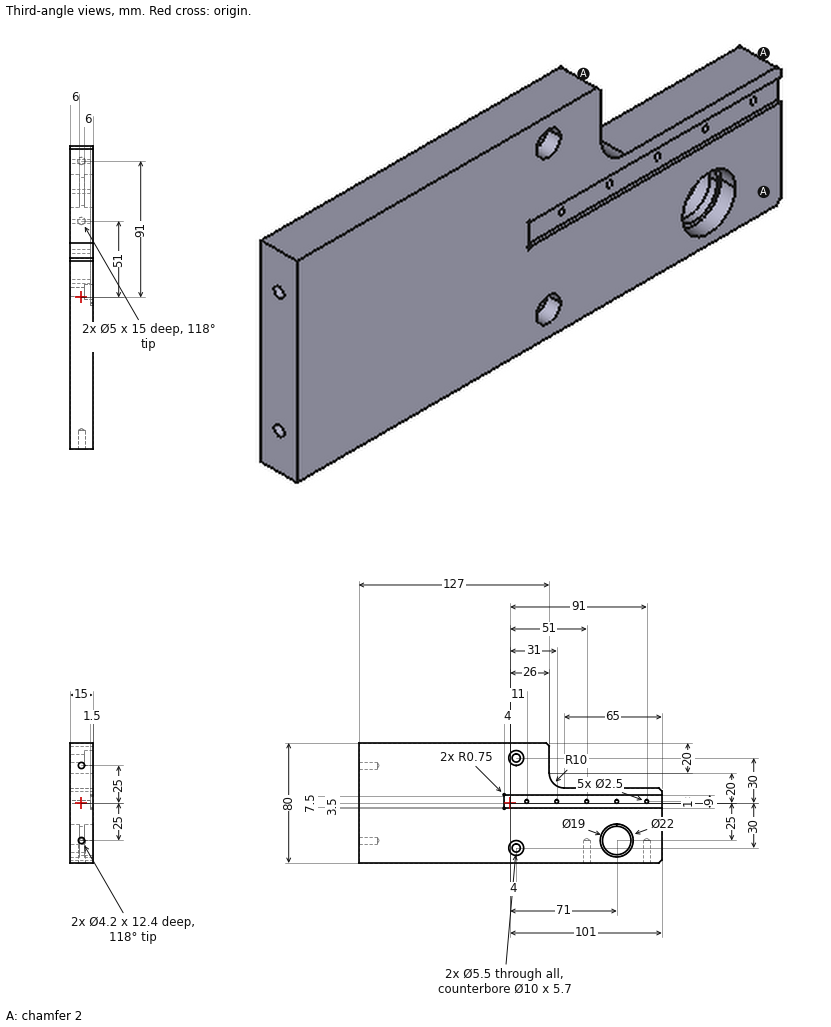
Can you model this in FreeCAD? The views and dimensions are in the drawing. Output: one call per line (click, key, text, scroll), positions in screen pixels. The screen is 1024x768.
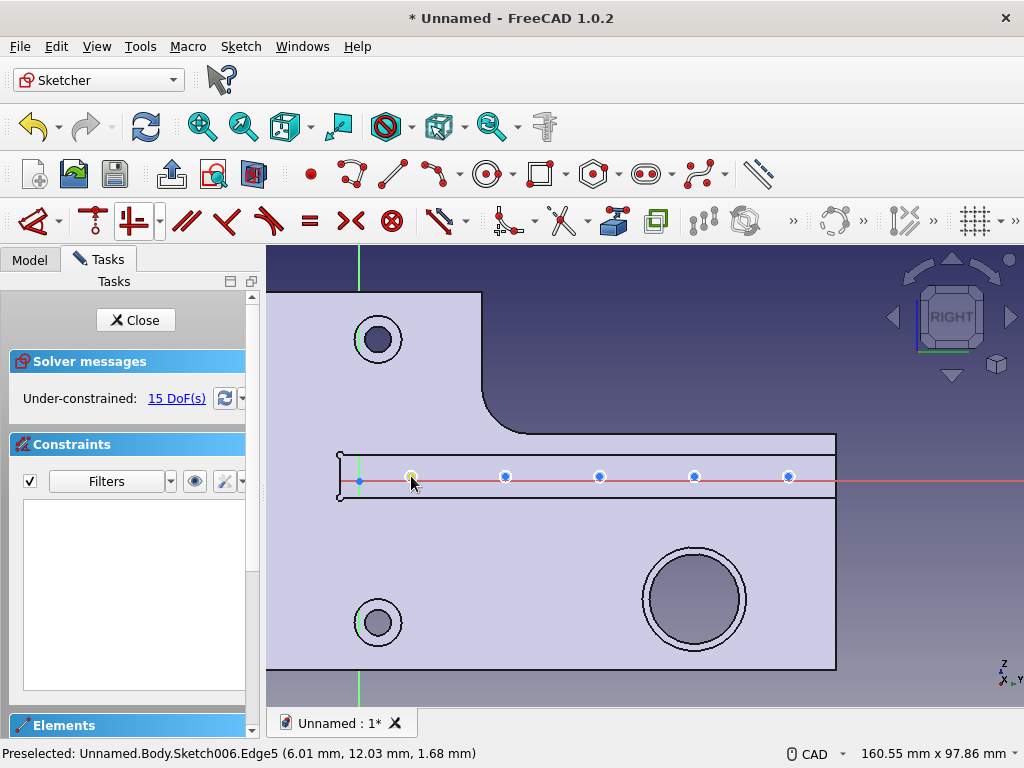
scroll(793, 472, up, 5)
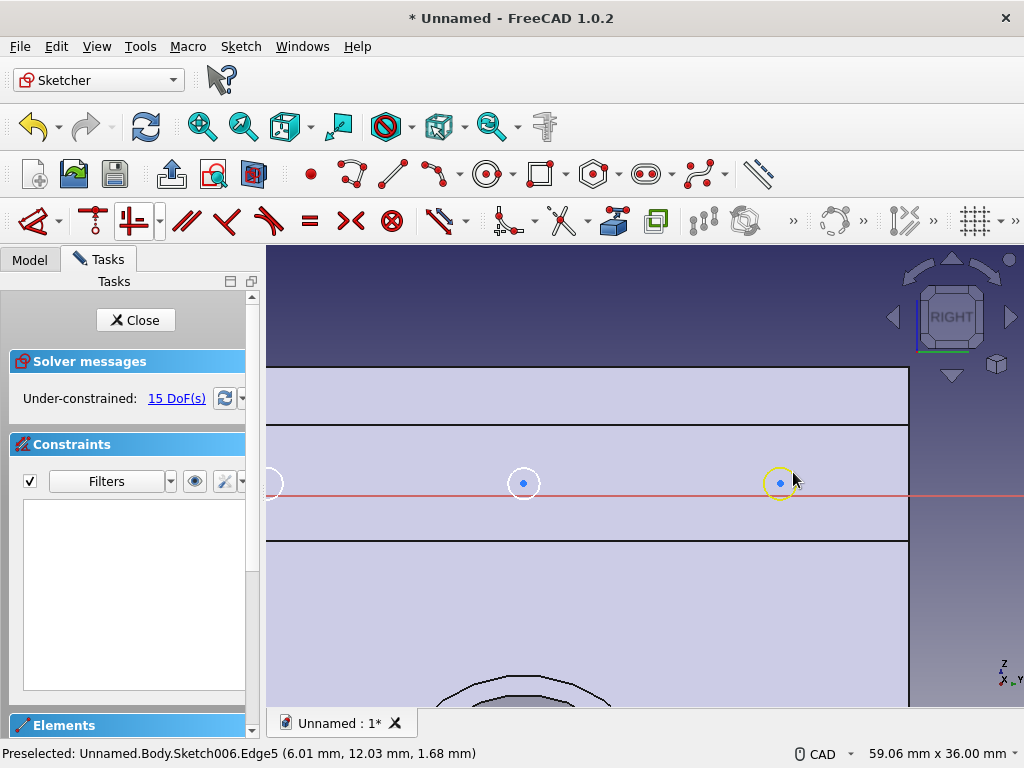
click(791, 472)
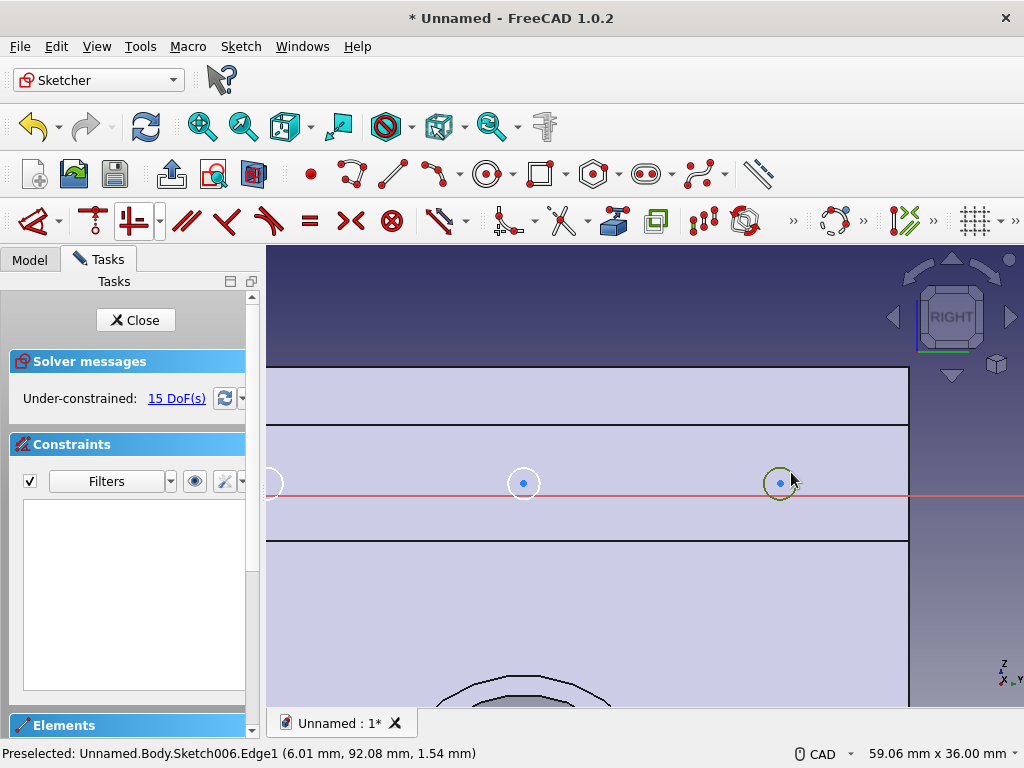
click(535, 473)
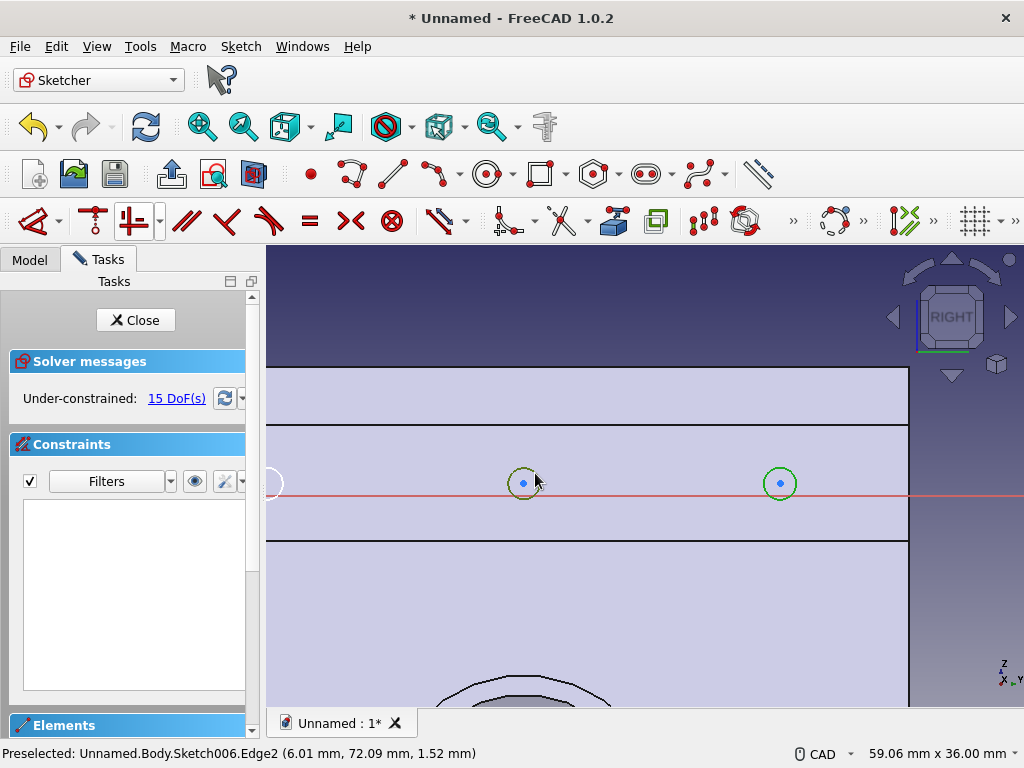
scroll(793, 472, down, 5)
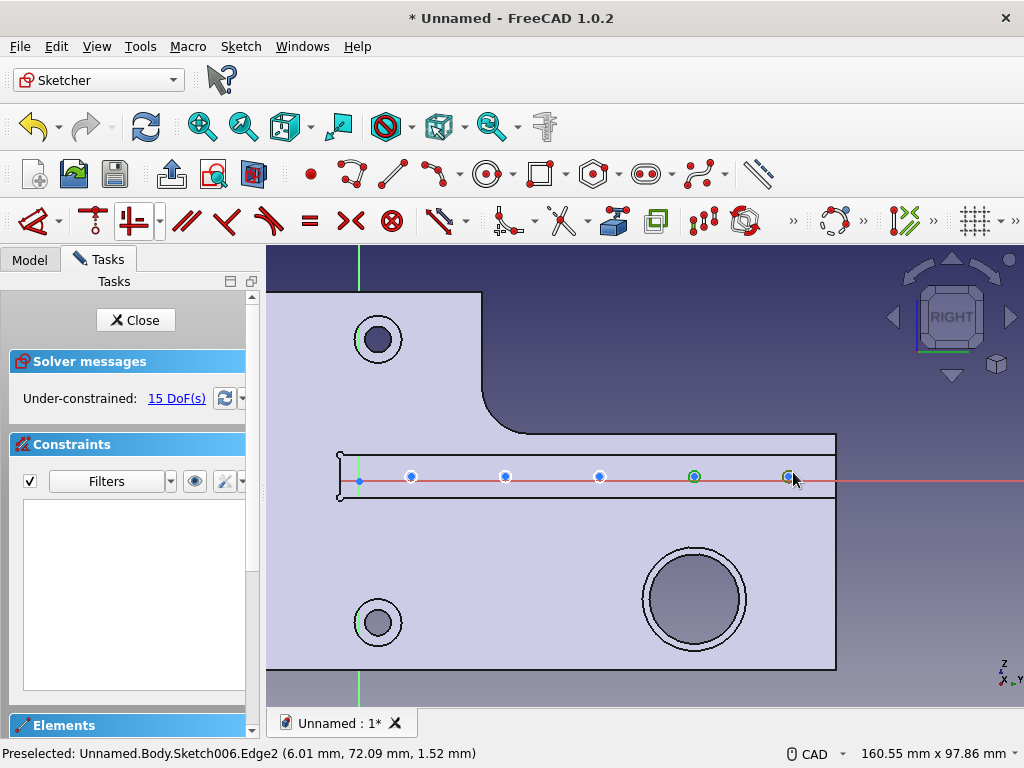
scroll(604, 472, up, 5)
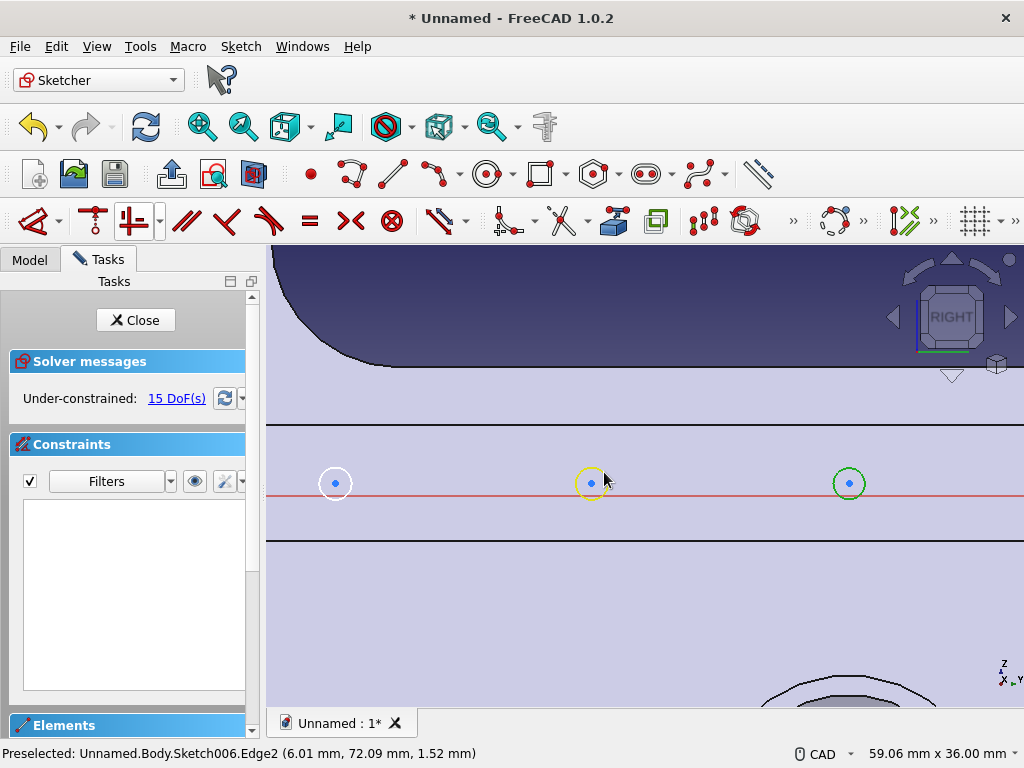
click(603, 472)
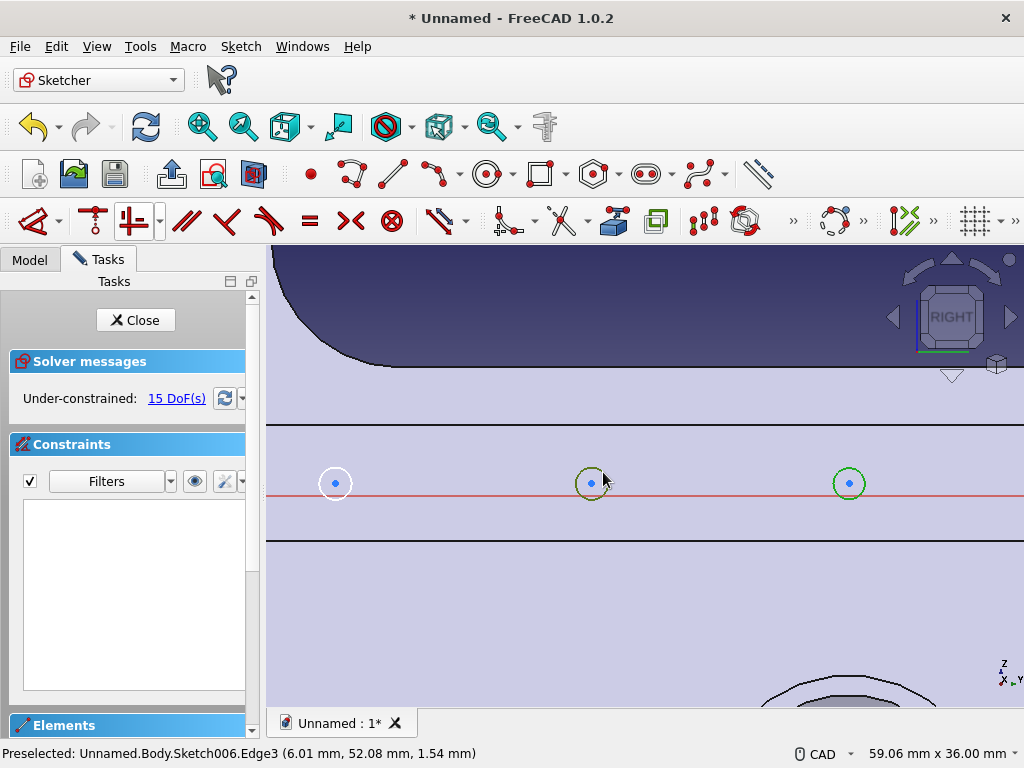
click(347, 472)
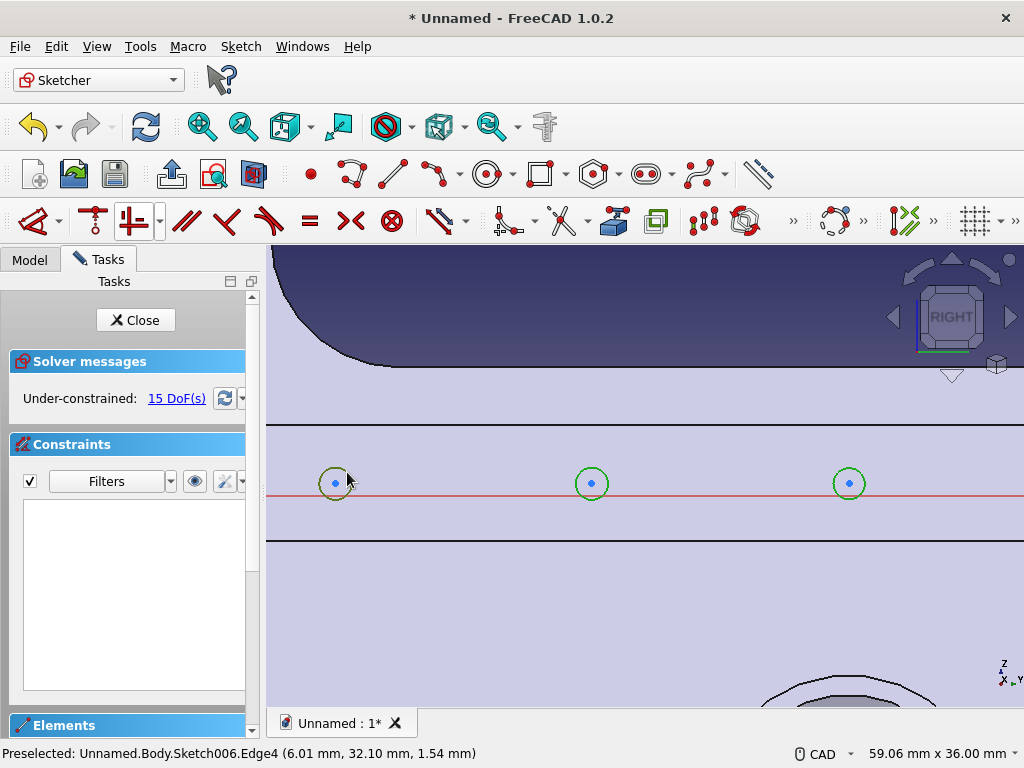
scroll(604, 472, down, 5)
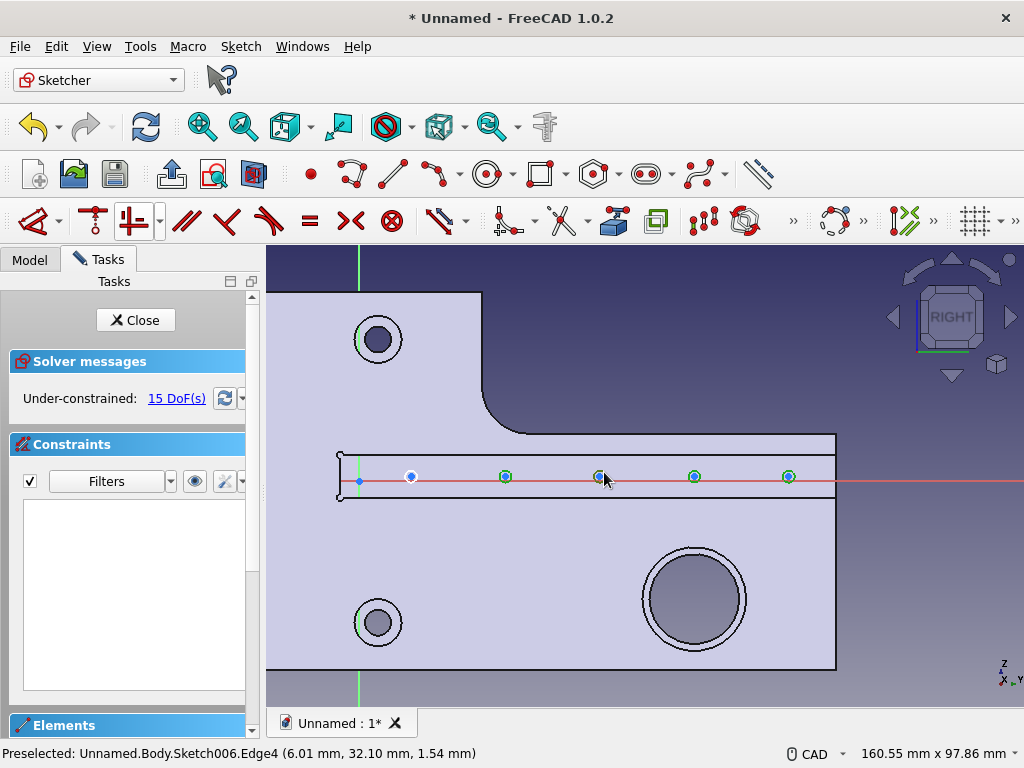
scroll(415, 472, up, 5)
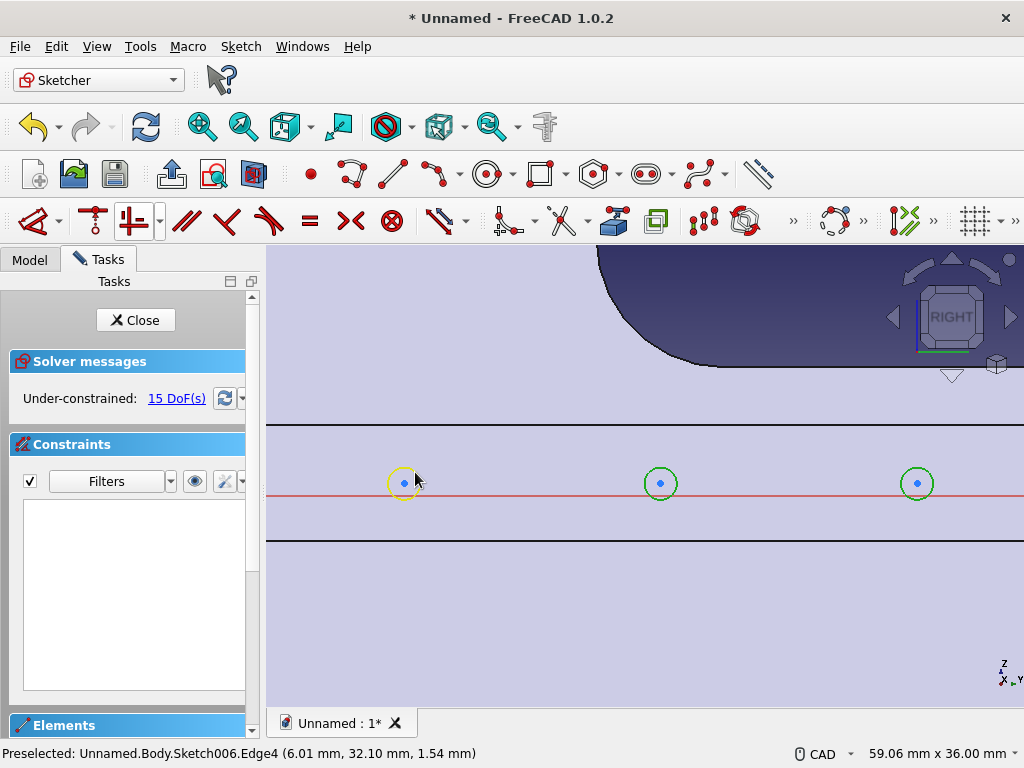
click(416, 472)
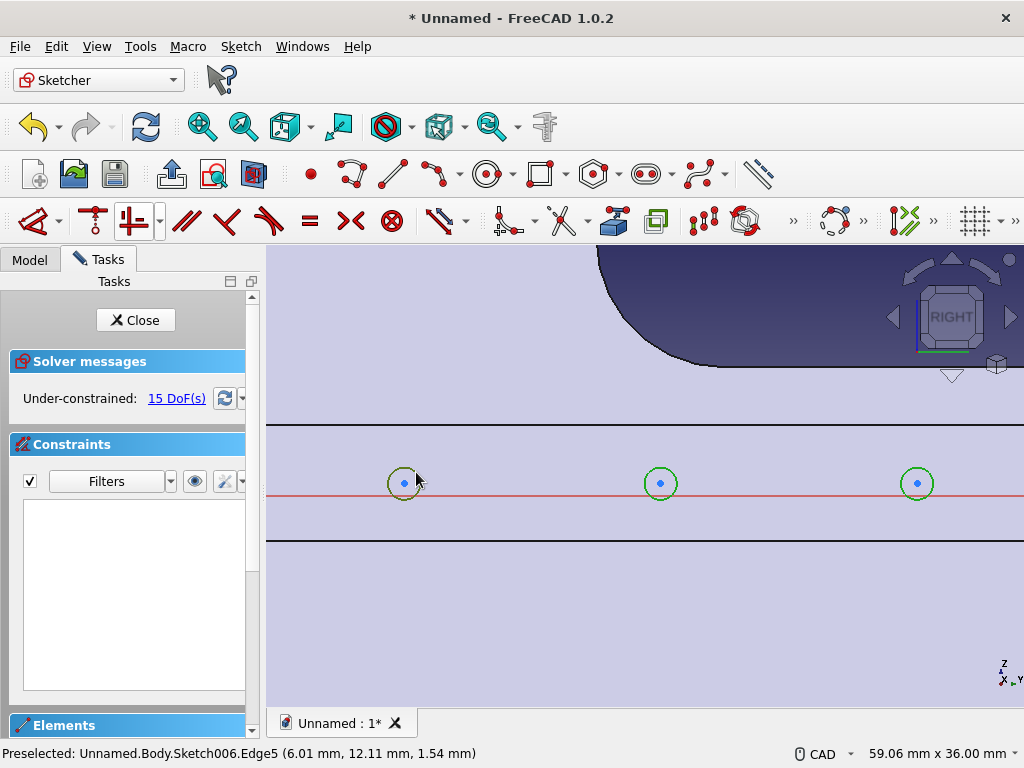
key(e)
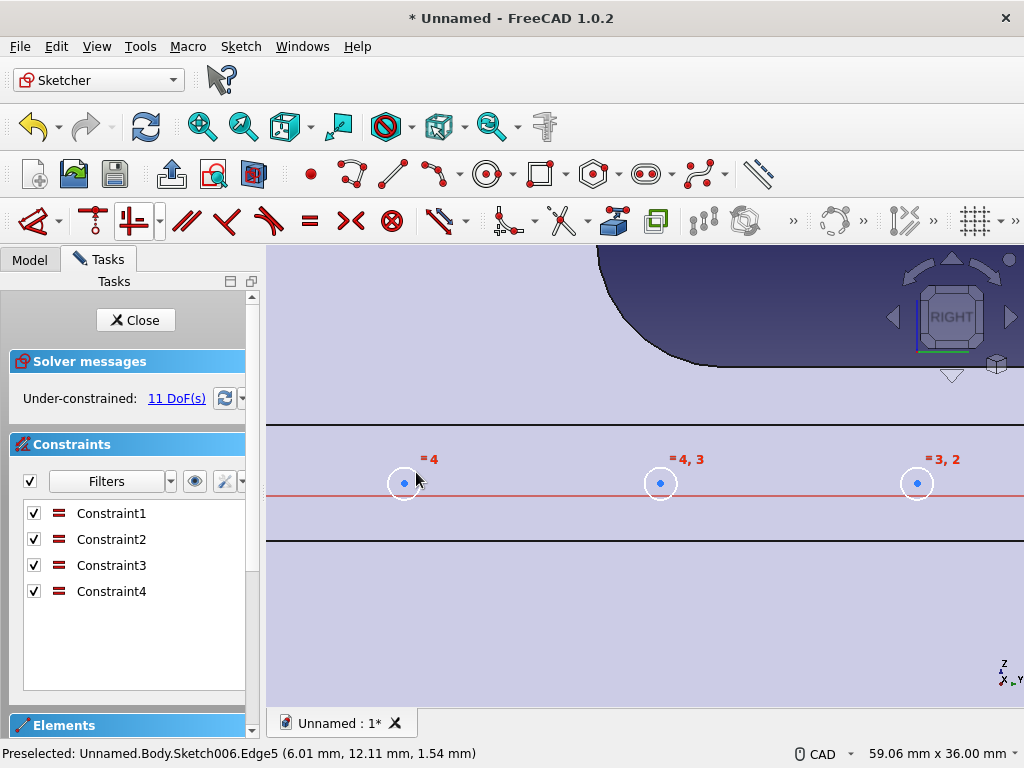
scroll(415, 472, down, 5)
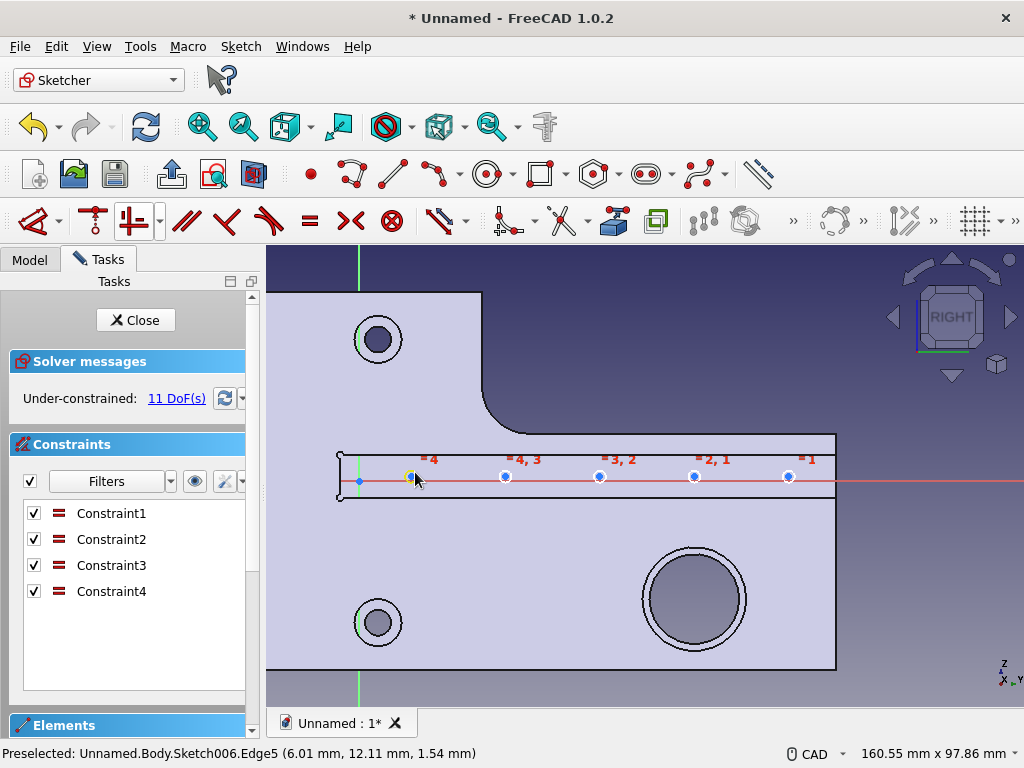
click(789, 477)